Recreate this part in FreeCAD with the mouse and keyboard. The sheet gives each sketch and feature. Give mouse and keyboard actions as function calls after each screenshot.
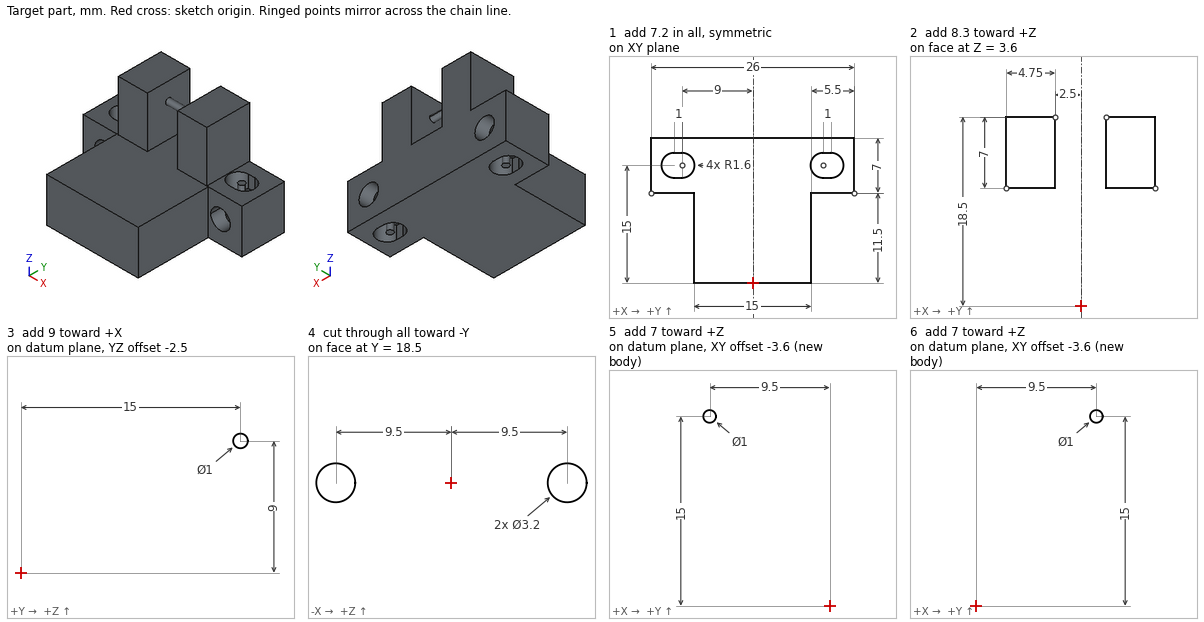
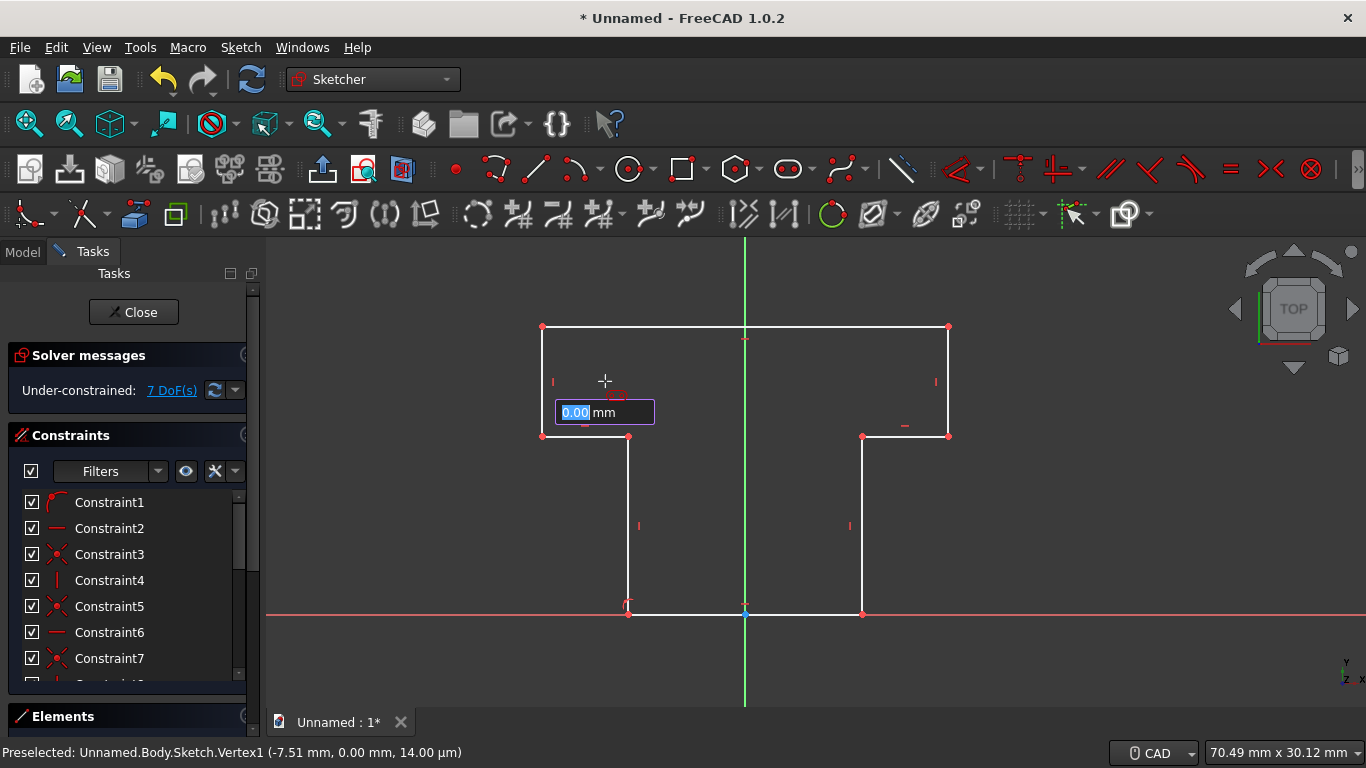
click(597, 356)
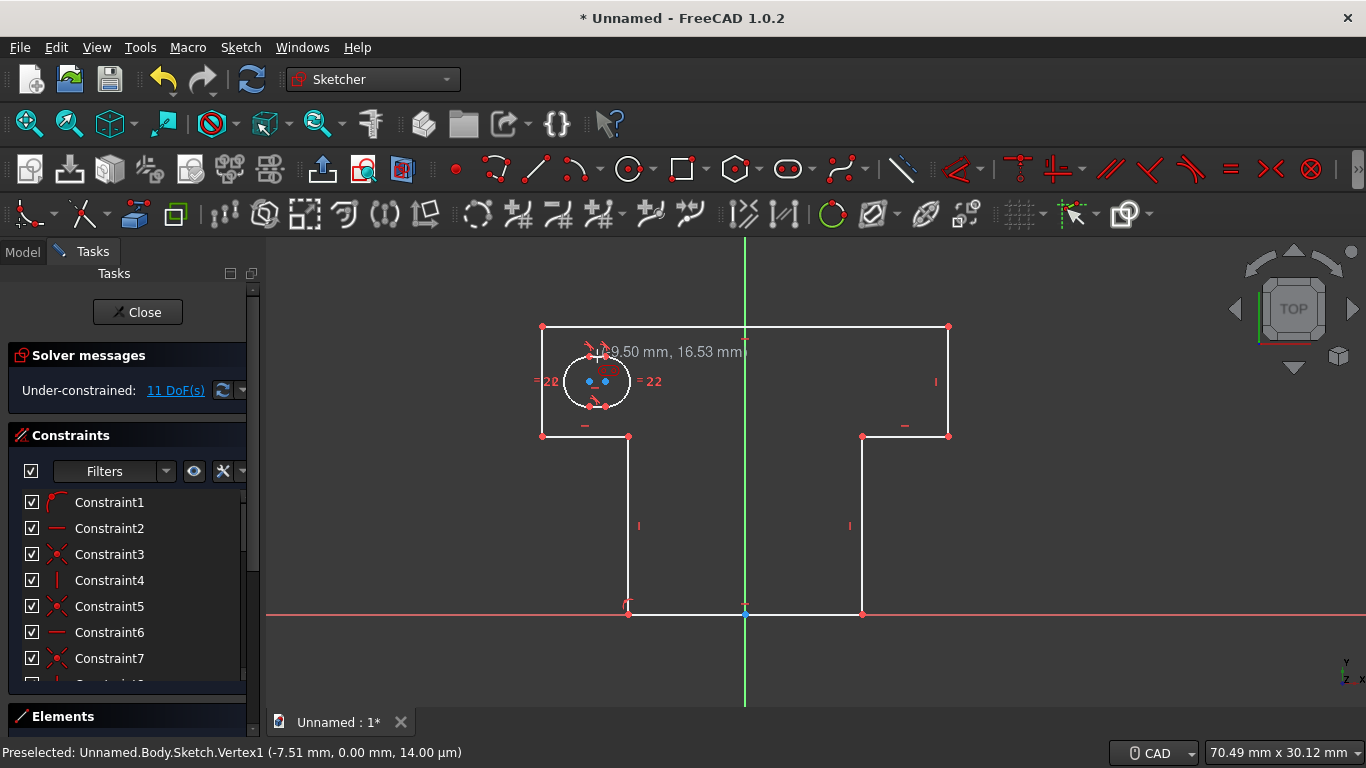
click(886, 381)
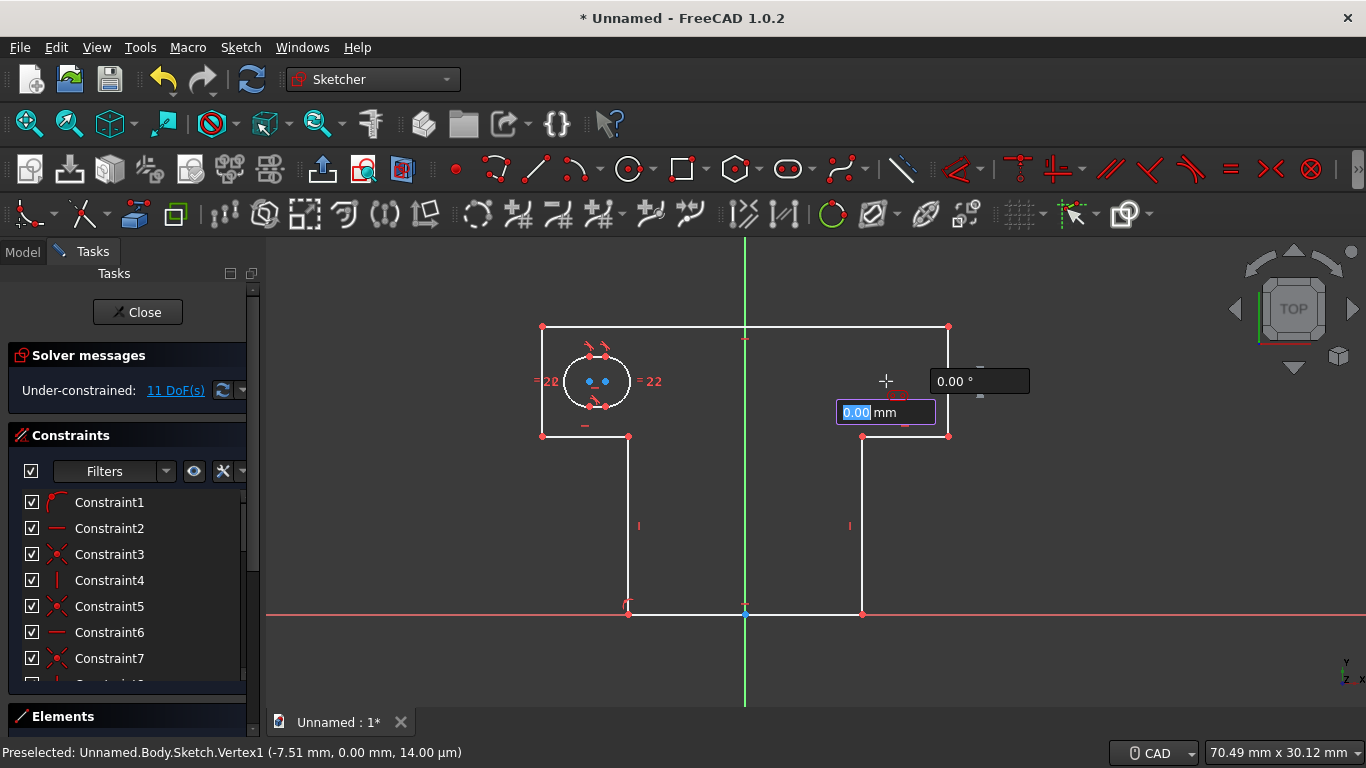
click(901, 381)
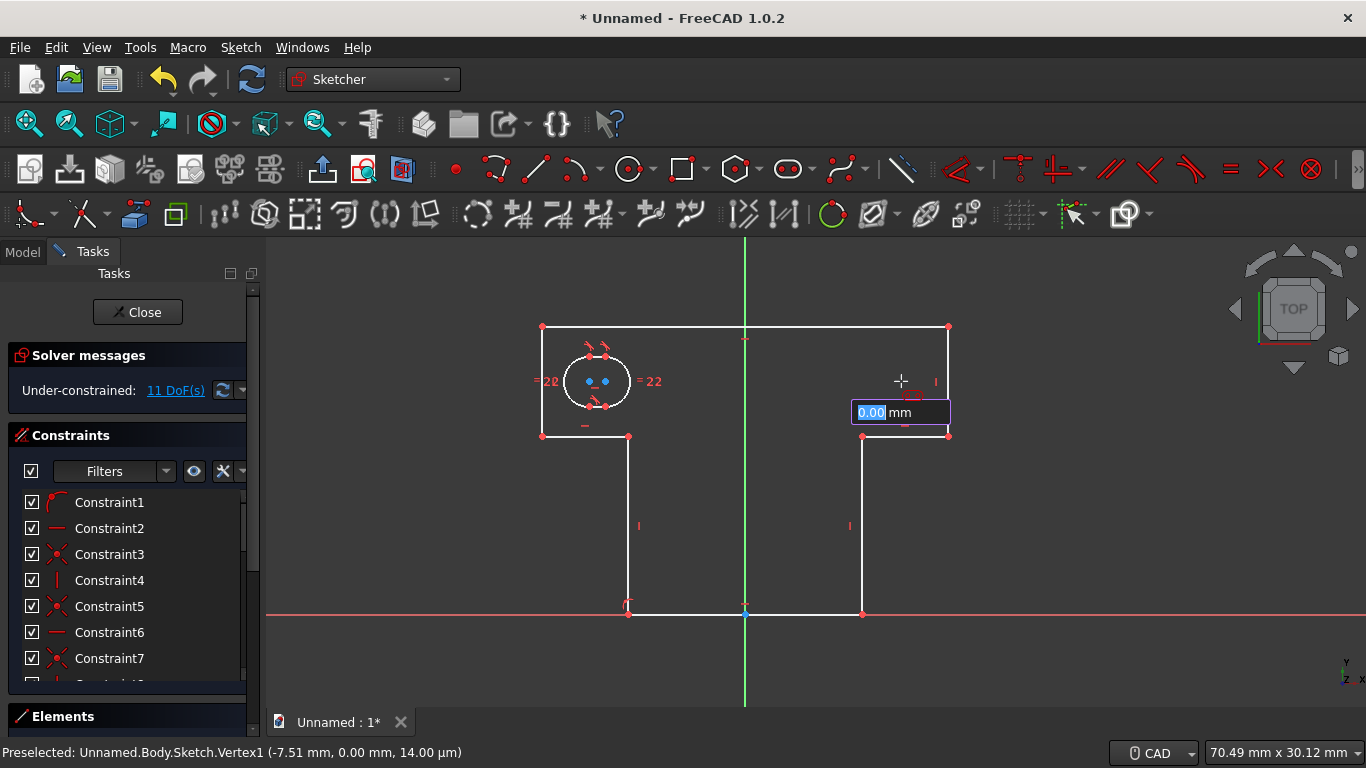
click(893, 356)
key(Escape)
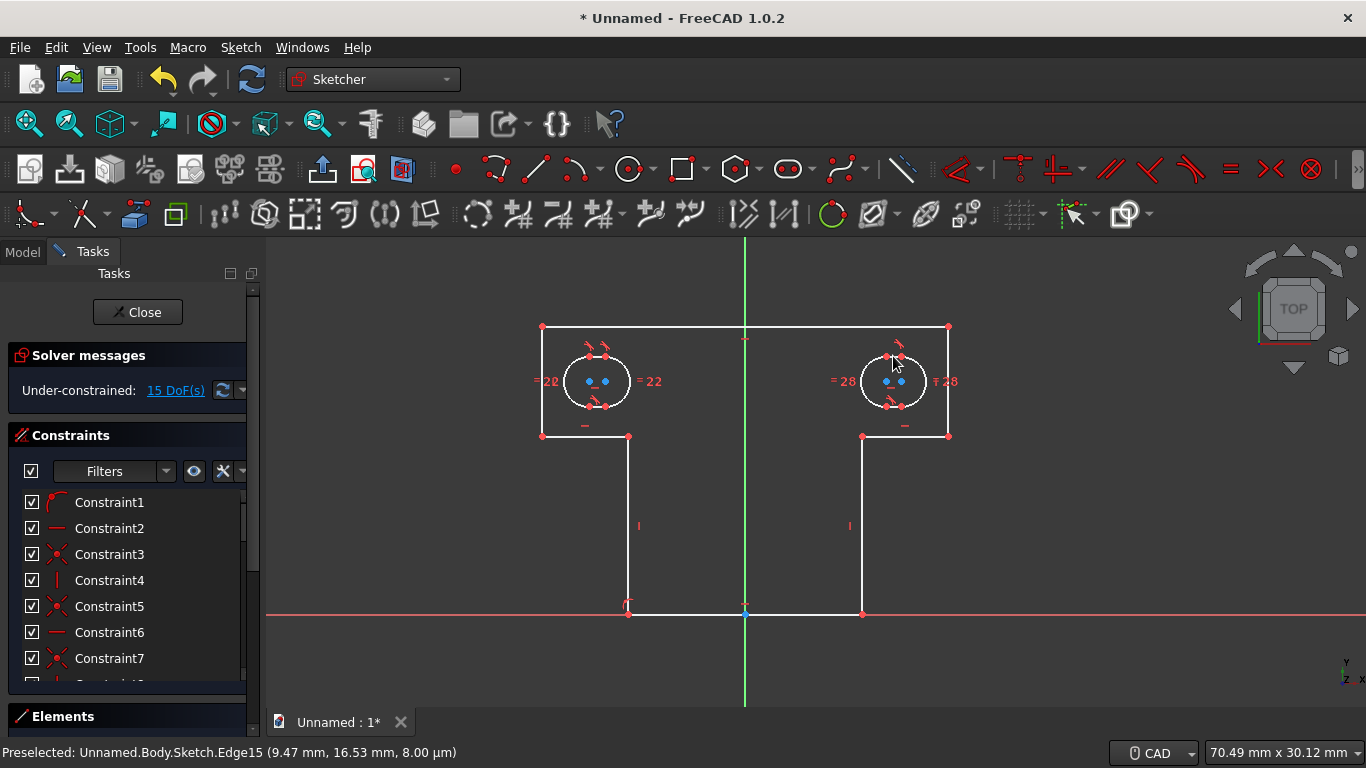
click(569, 367)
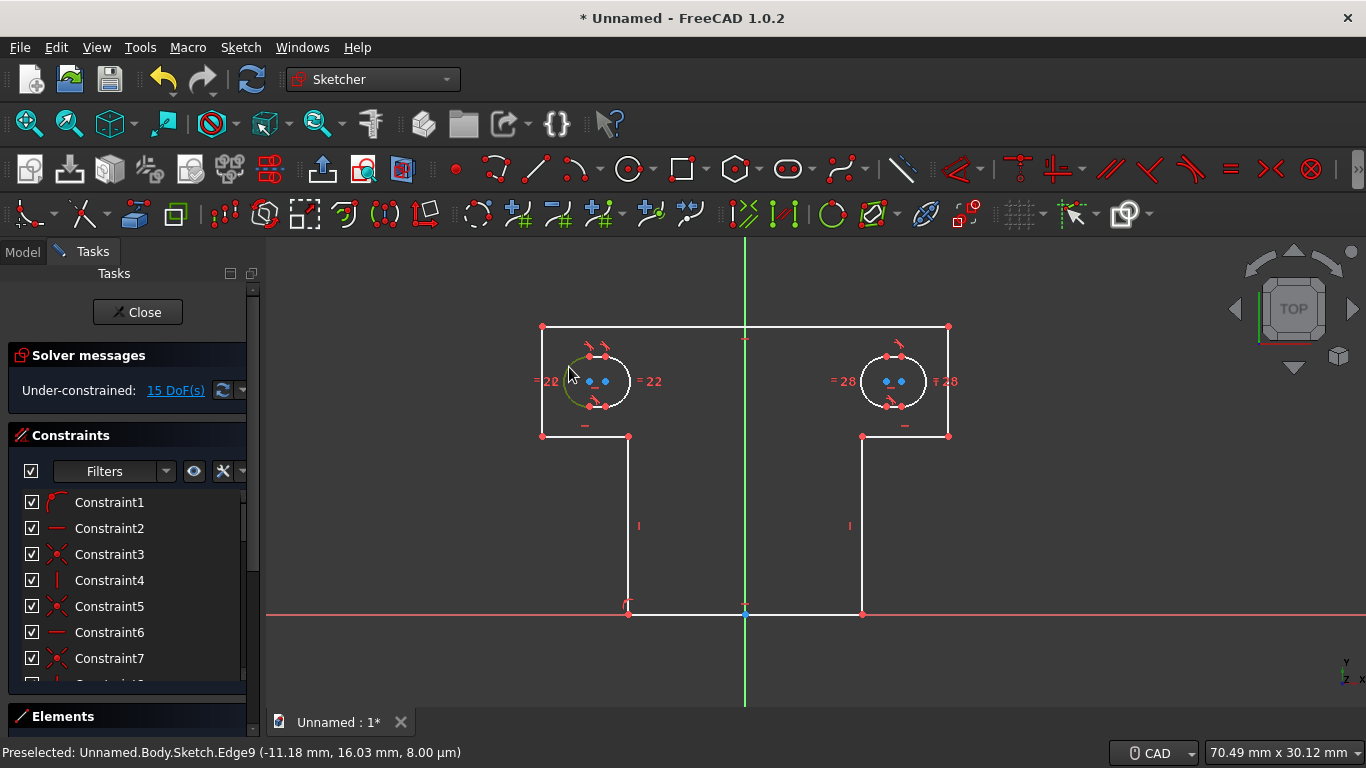
click(866, 367)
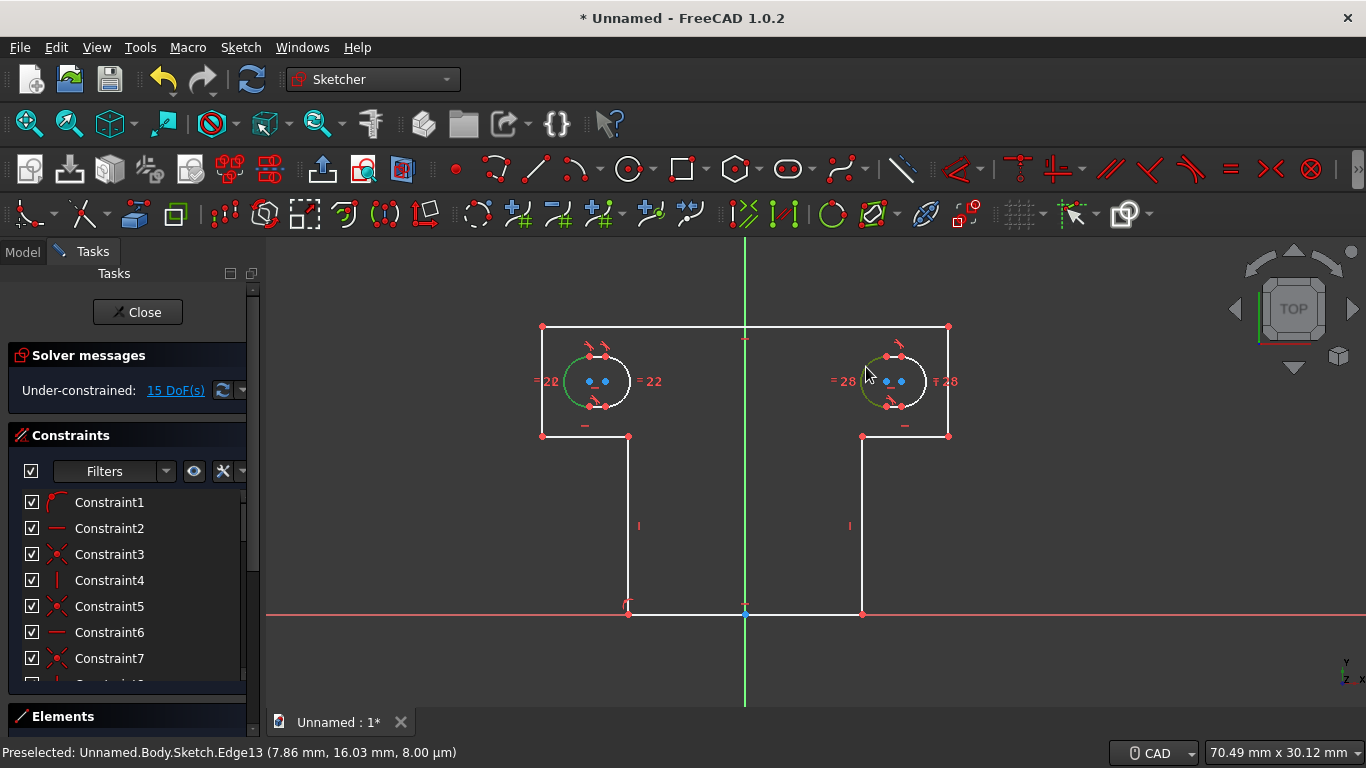
click(1232, 170)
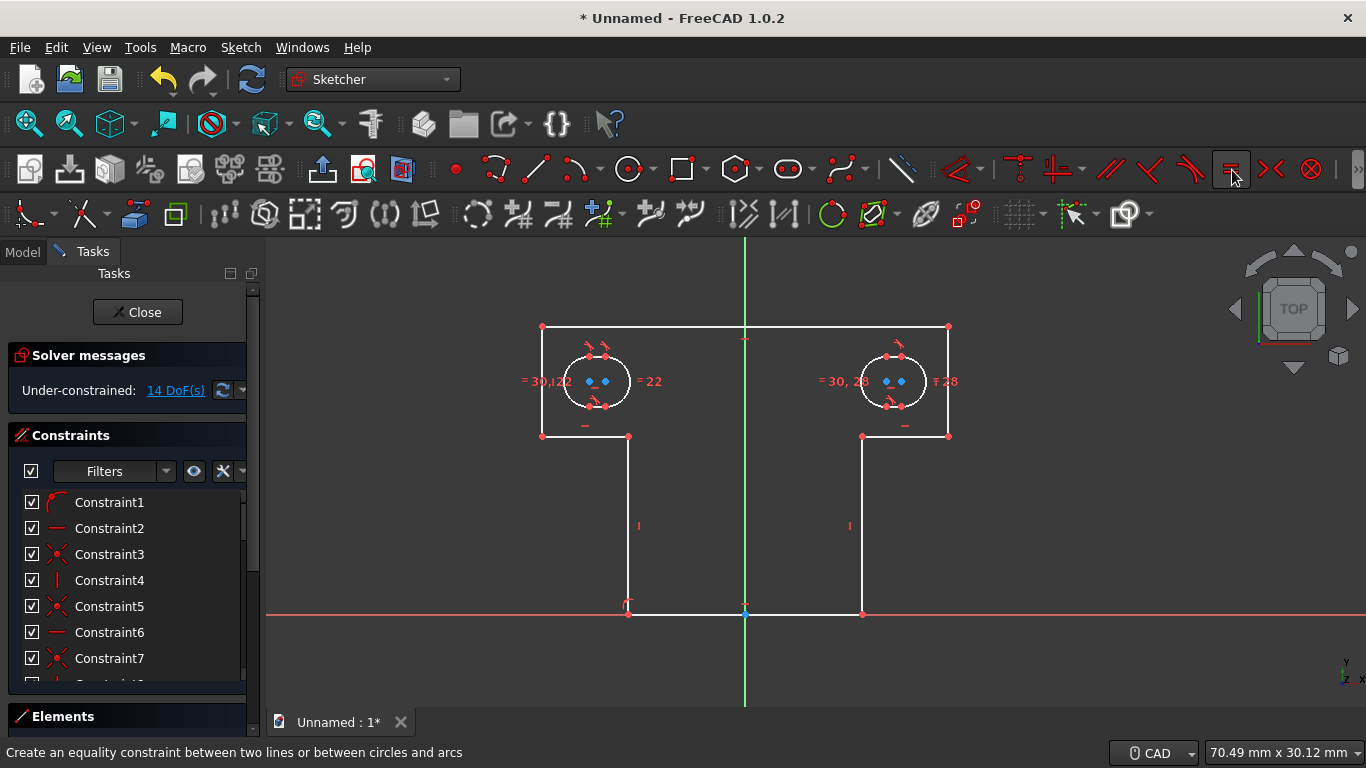
click(605, 382)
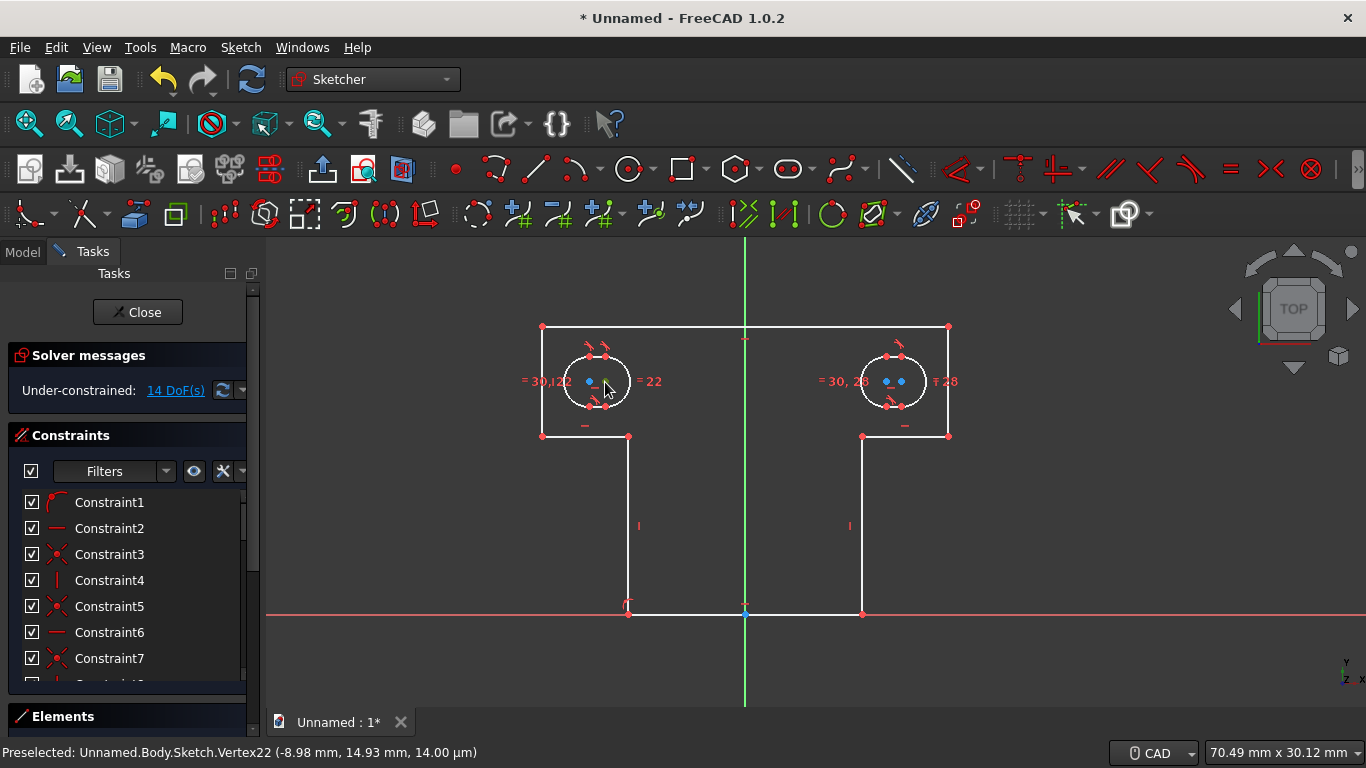
click(886, 382)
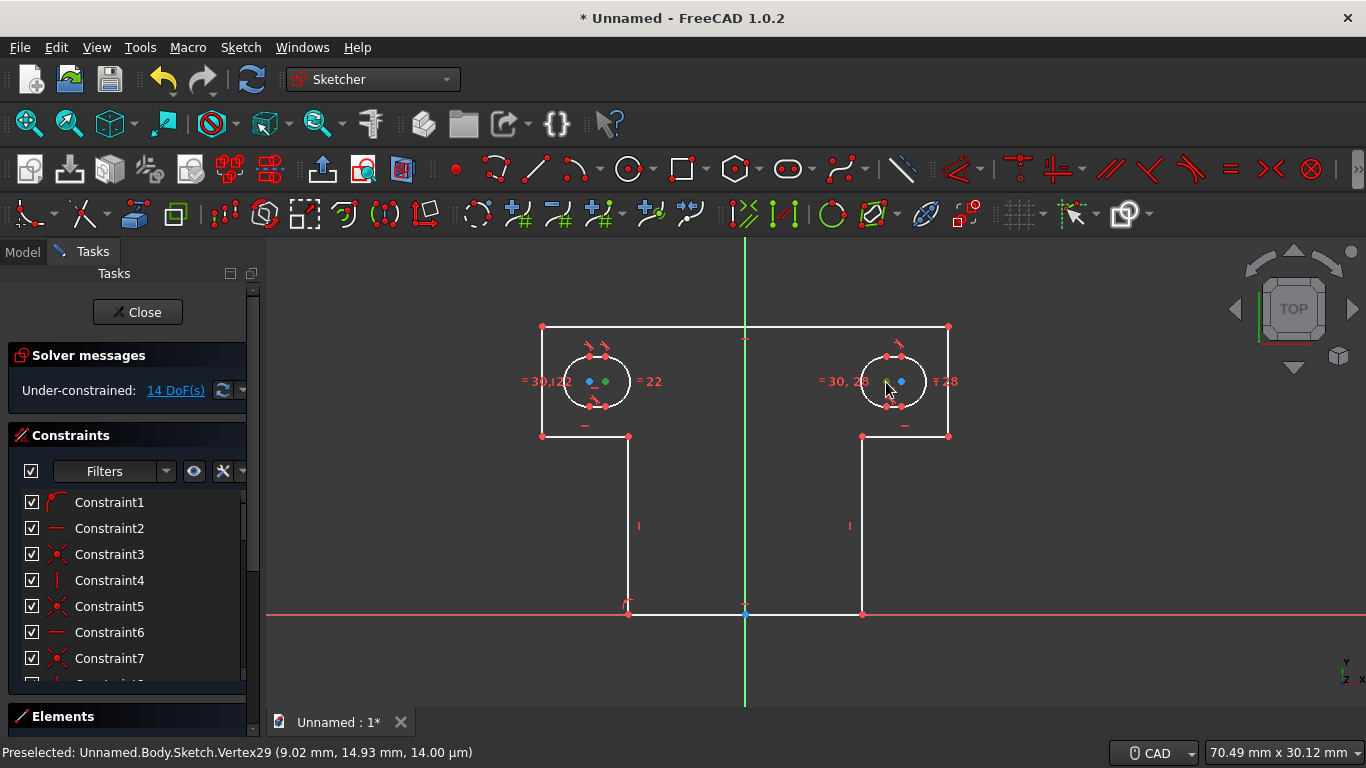
click(745, 649)